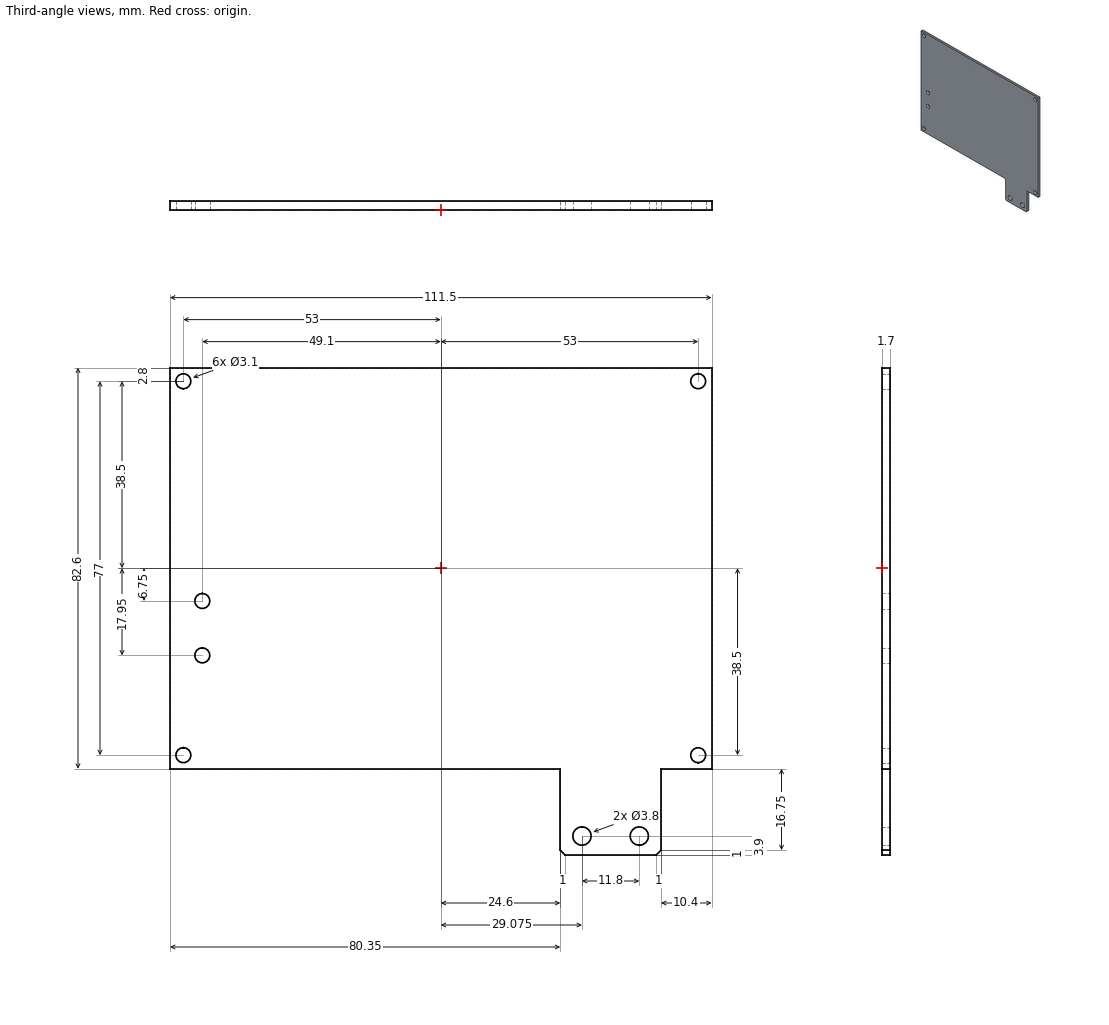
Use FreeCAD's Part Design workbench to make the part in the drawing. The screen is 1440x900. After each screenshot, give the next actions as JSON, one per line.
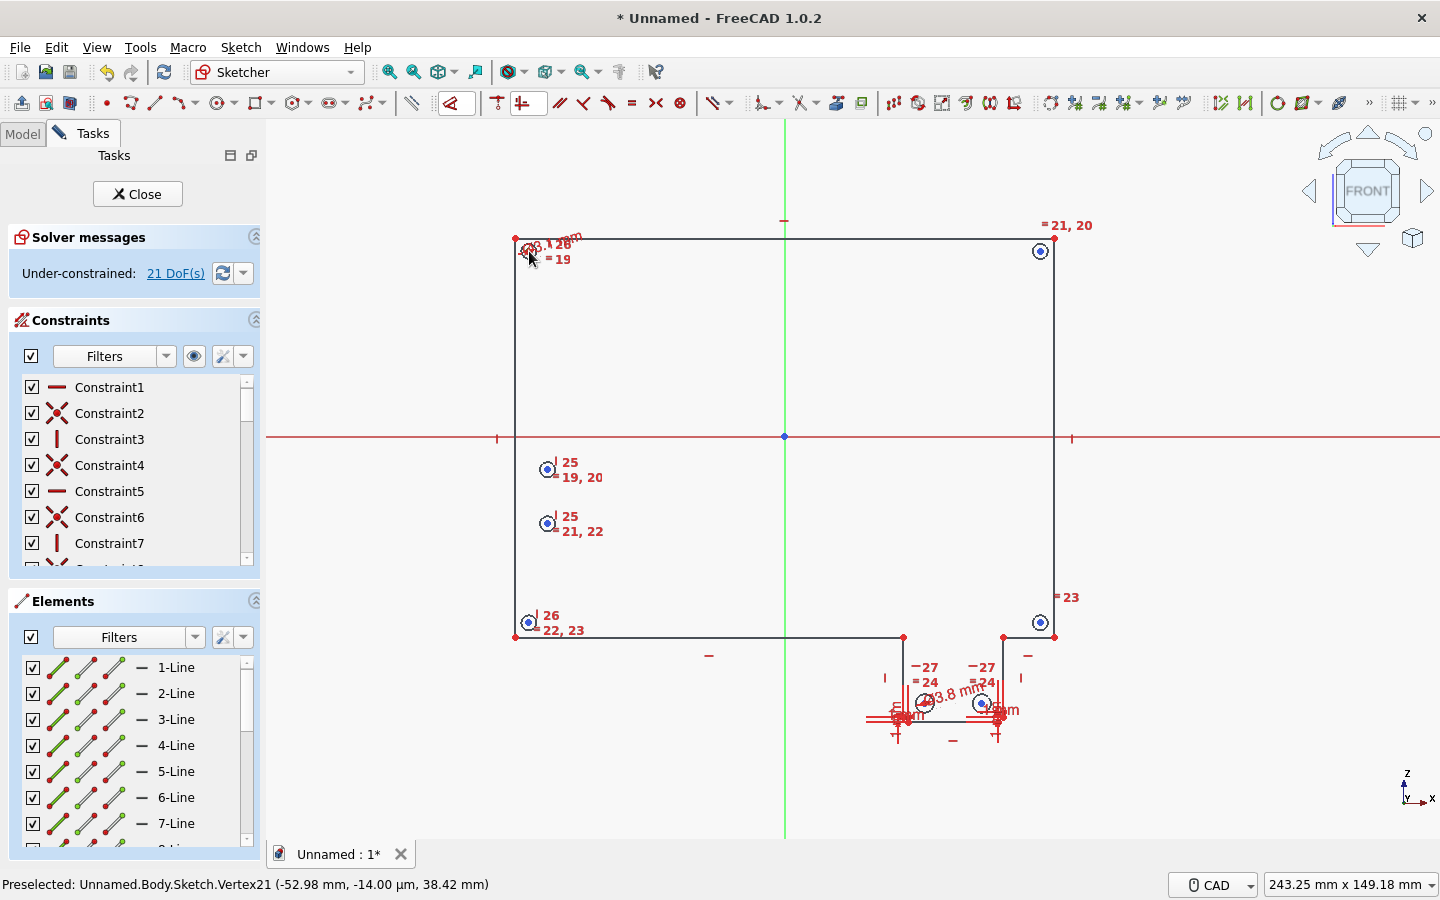
{"action": "key", "text": "l"}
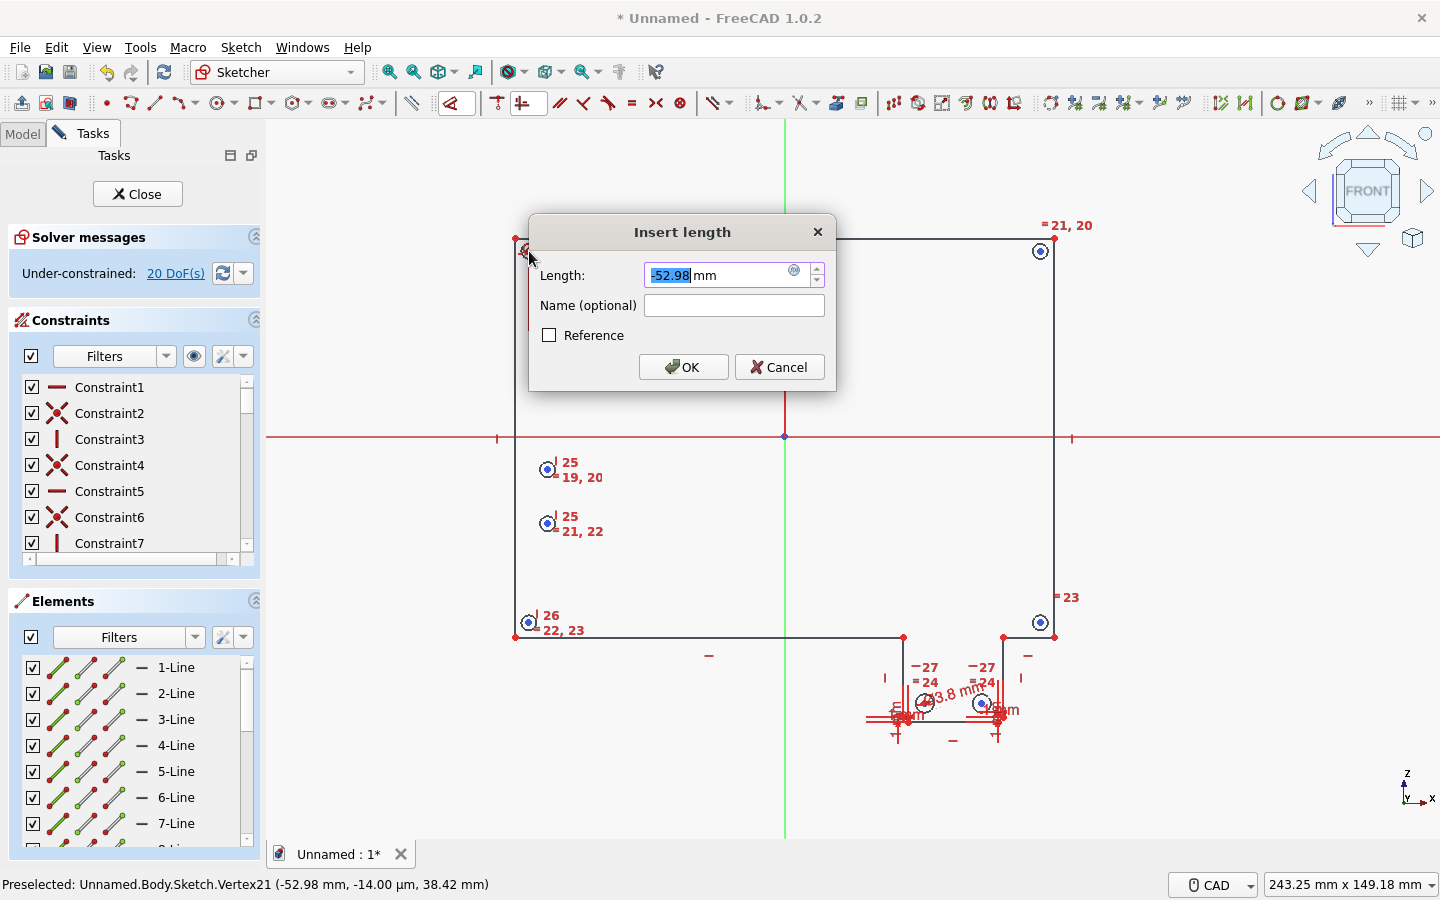
{"action": "type", "text": "-53"}
{"action": "key", "text": "Return"}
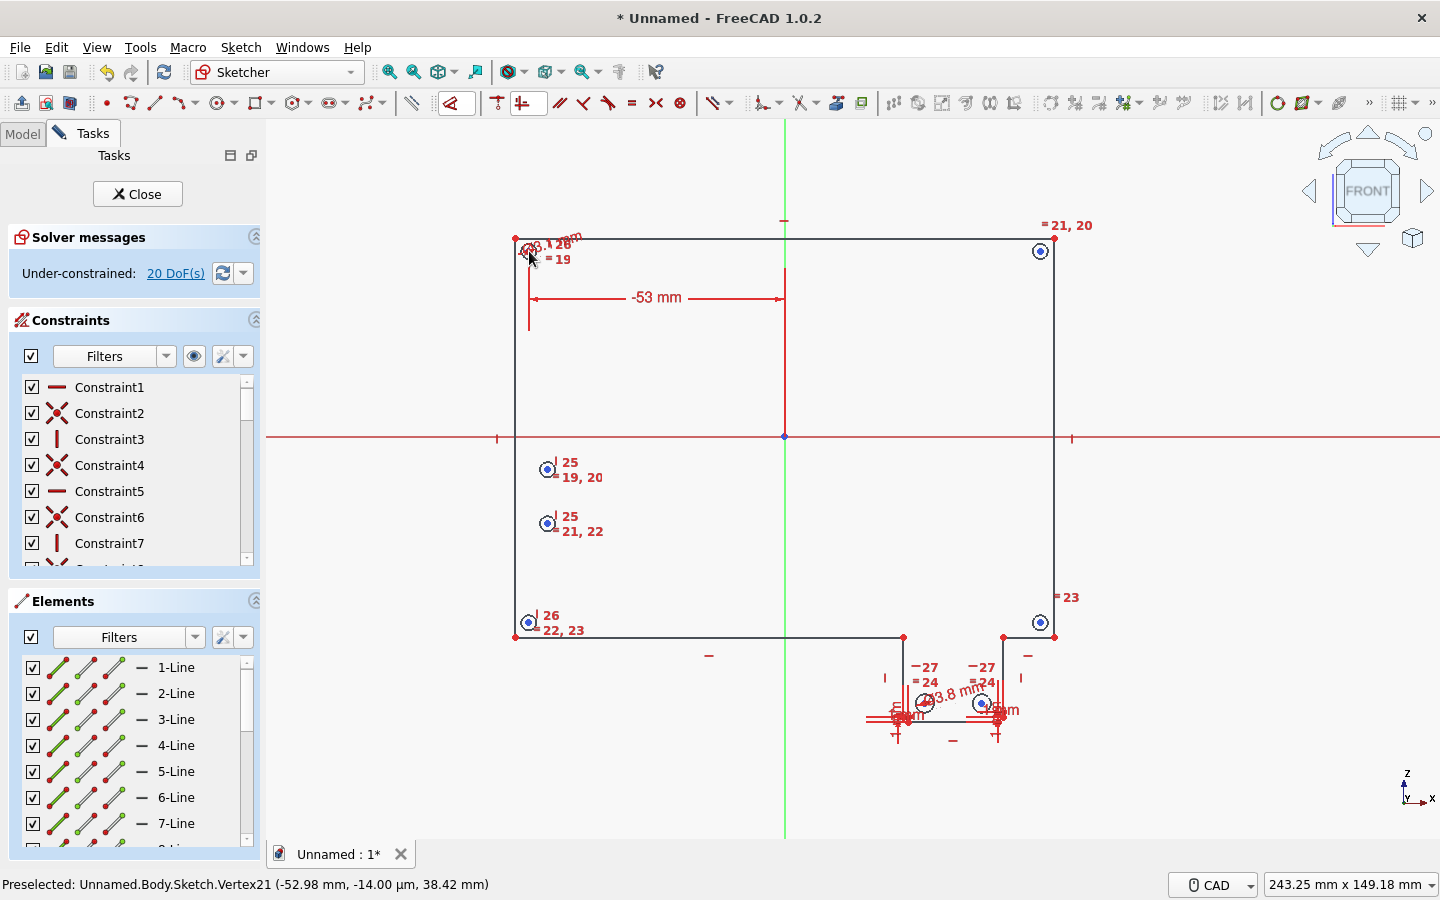
{"action": "left_click", "coordinate": [1040, 251]}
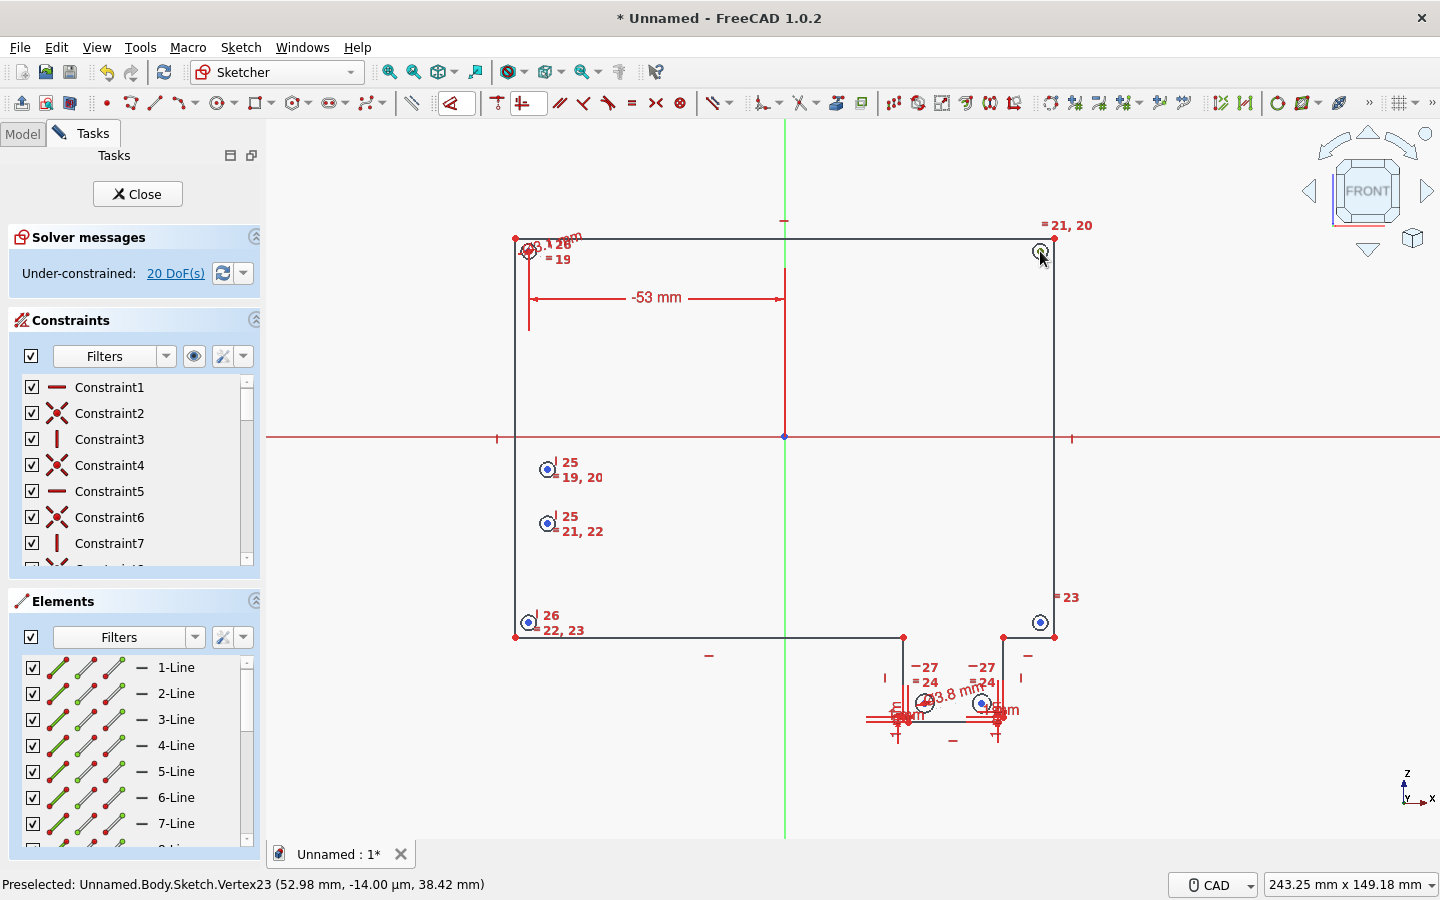
{"action": "key", "text": "l"}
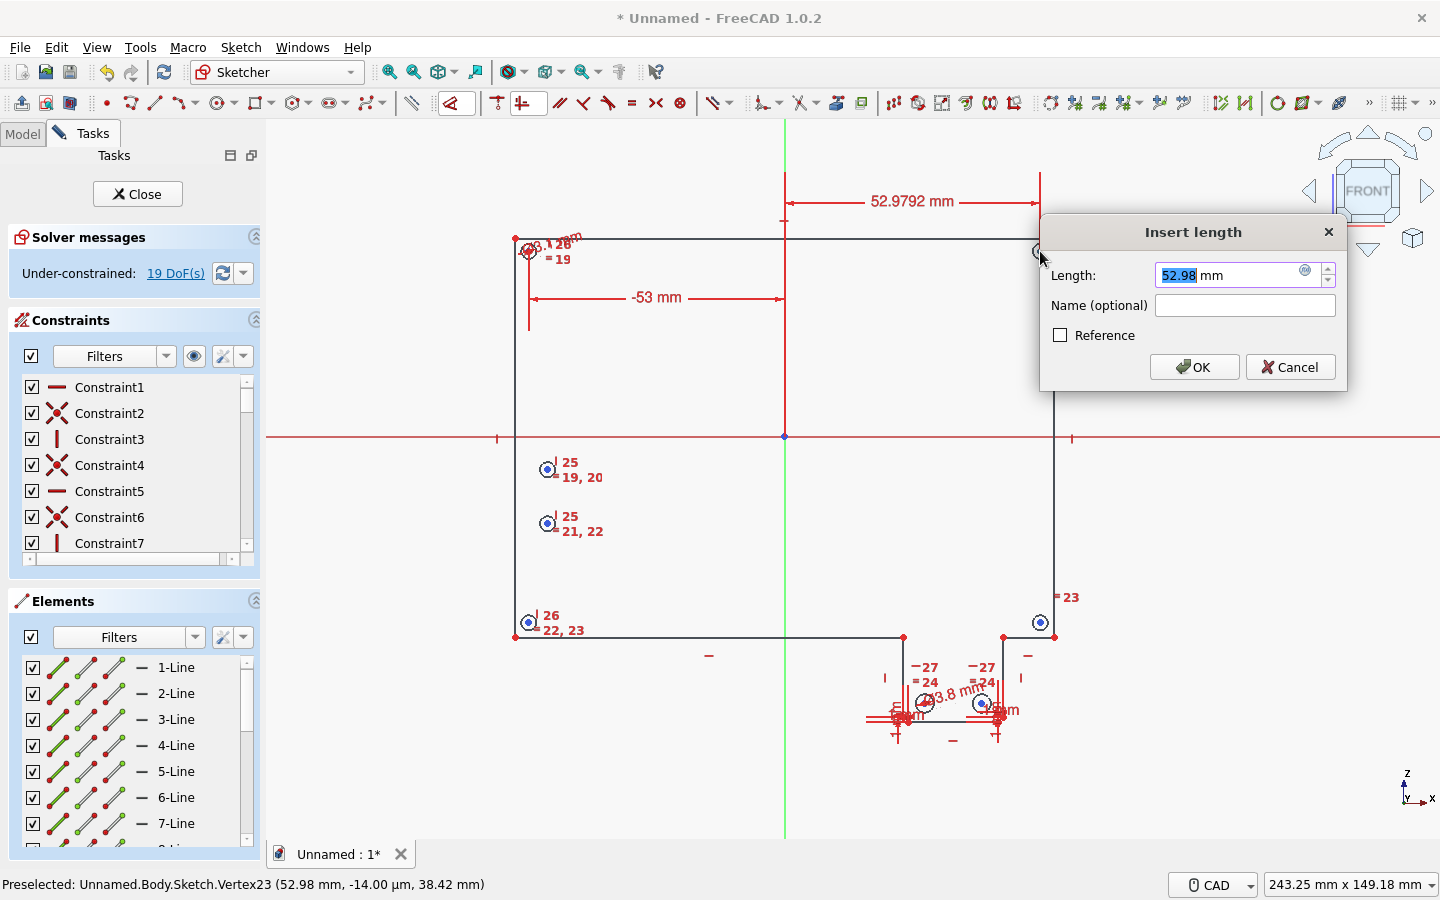
{"action": "type", "text": "53"}
{"action": "key", "text": "Return"}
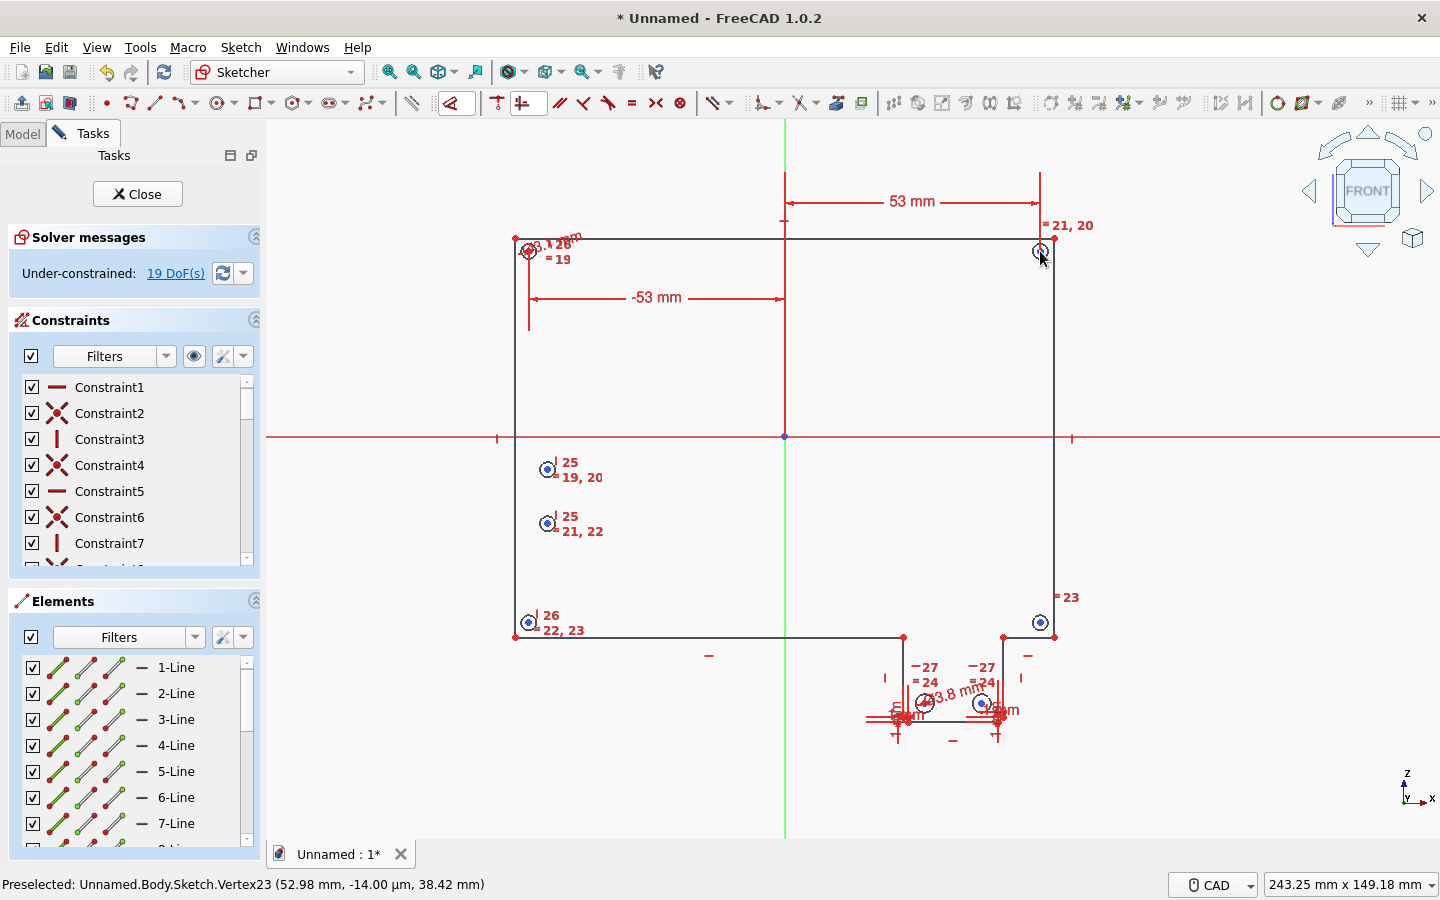
{"action": "left_click", "coordinate": [1040, 623]}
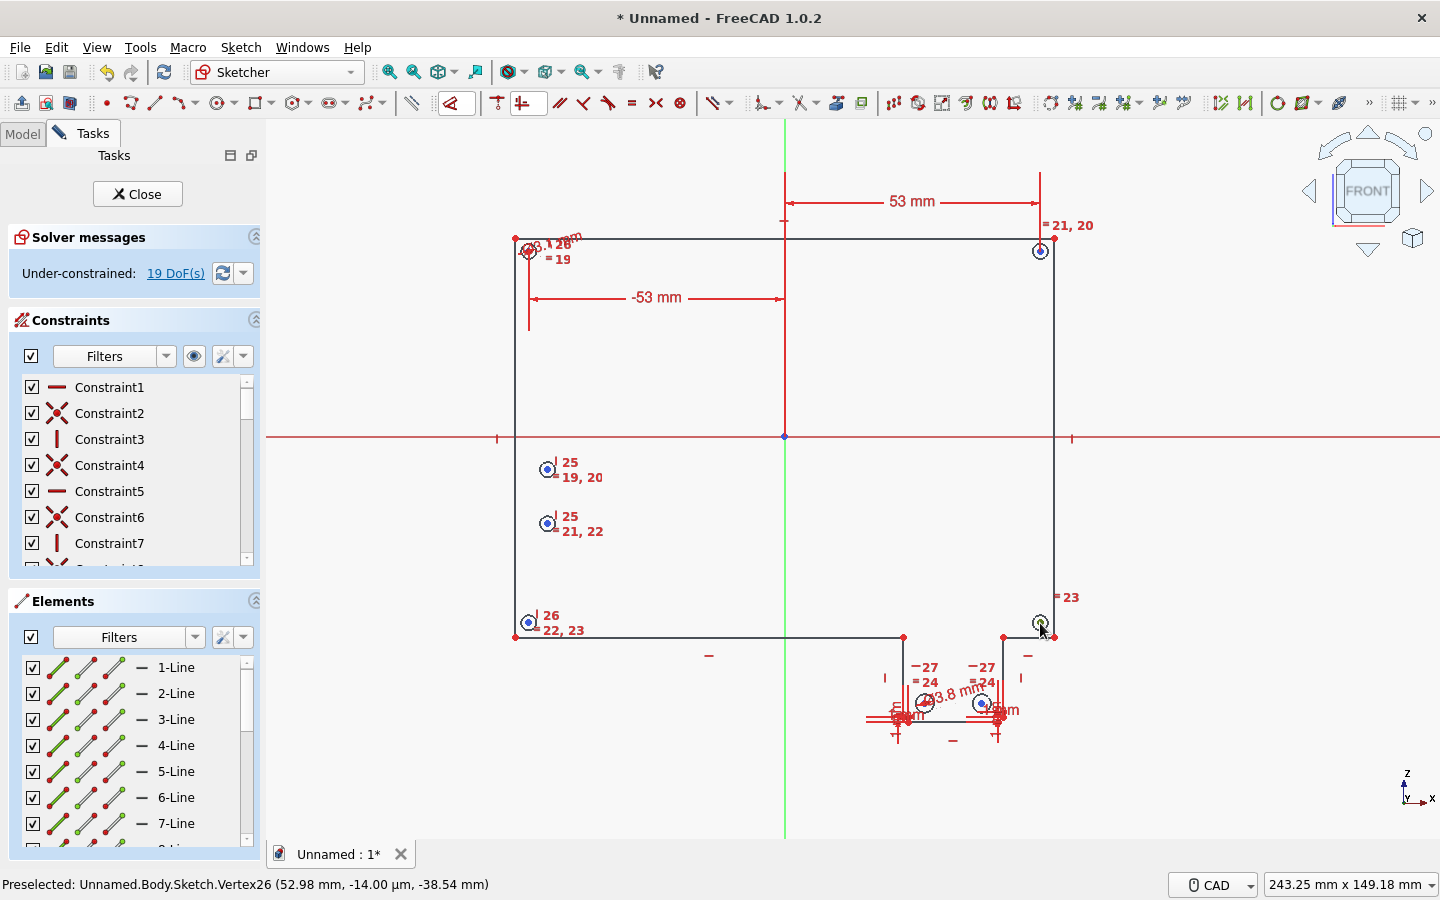
{"action": "key", "text": "l"}